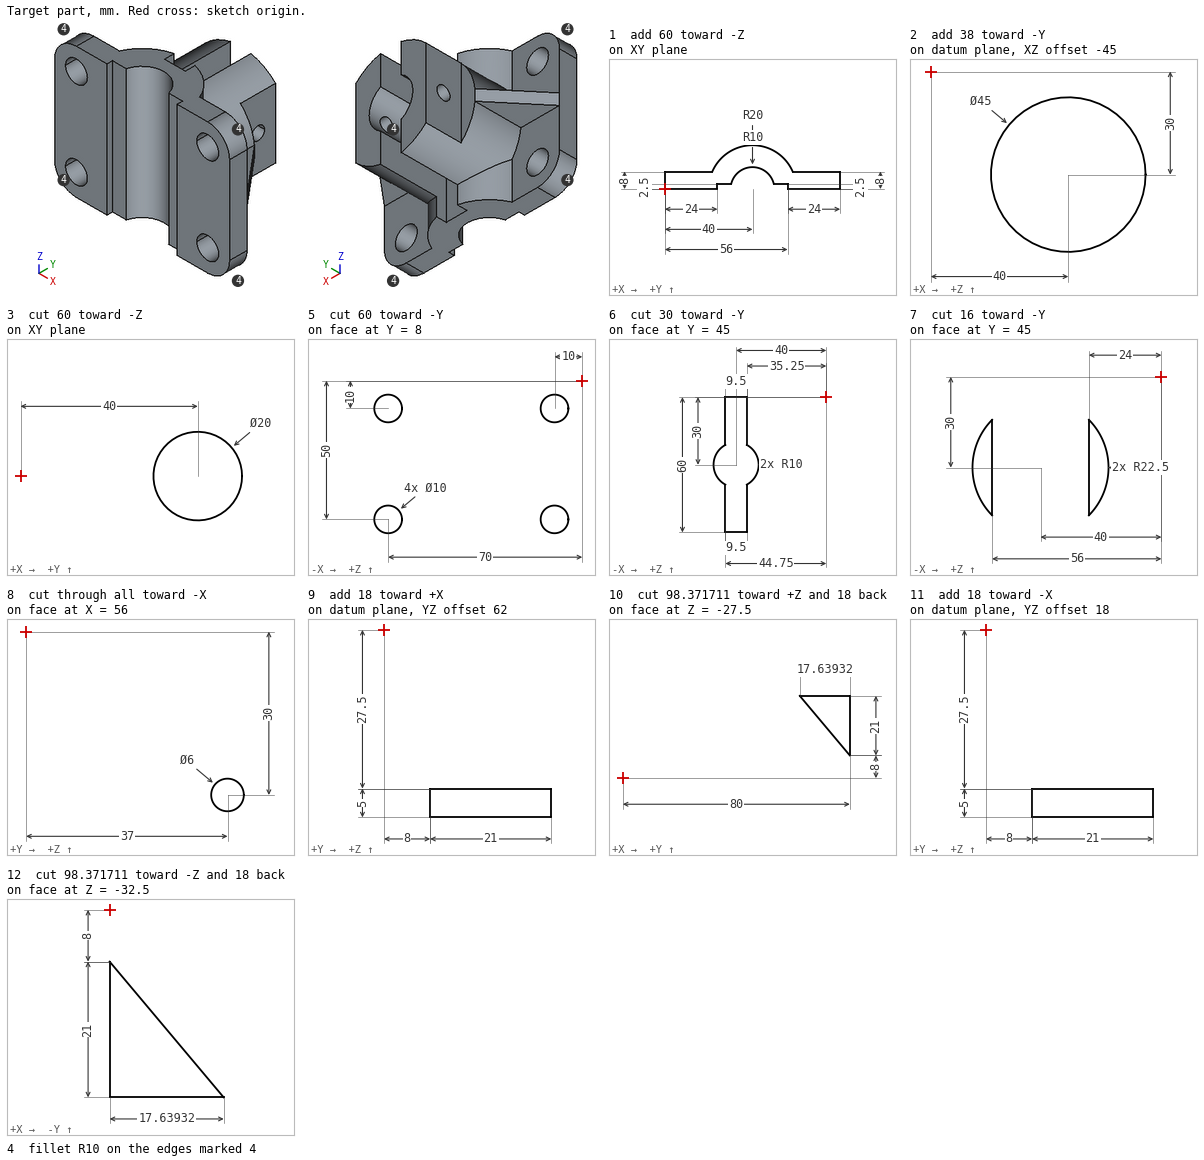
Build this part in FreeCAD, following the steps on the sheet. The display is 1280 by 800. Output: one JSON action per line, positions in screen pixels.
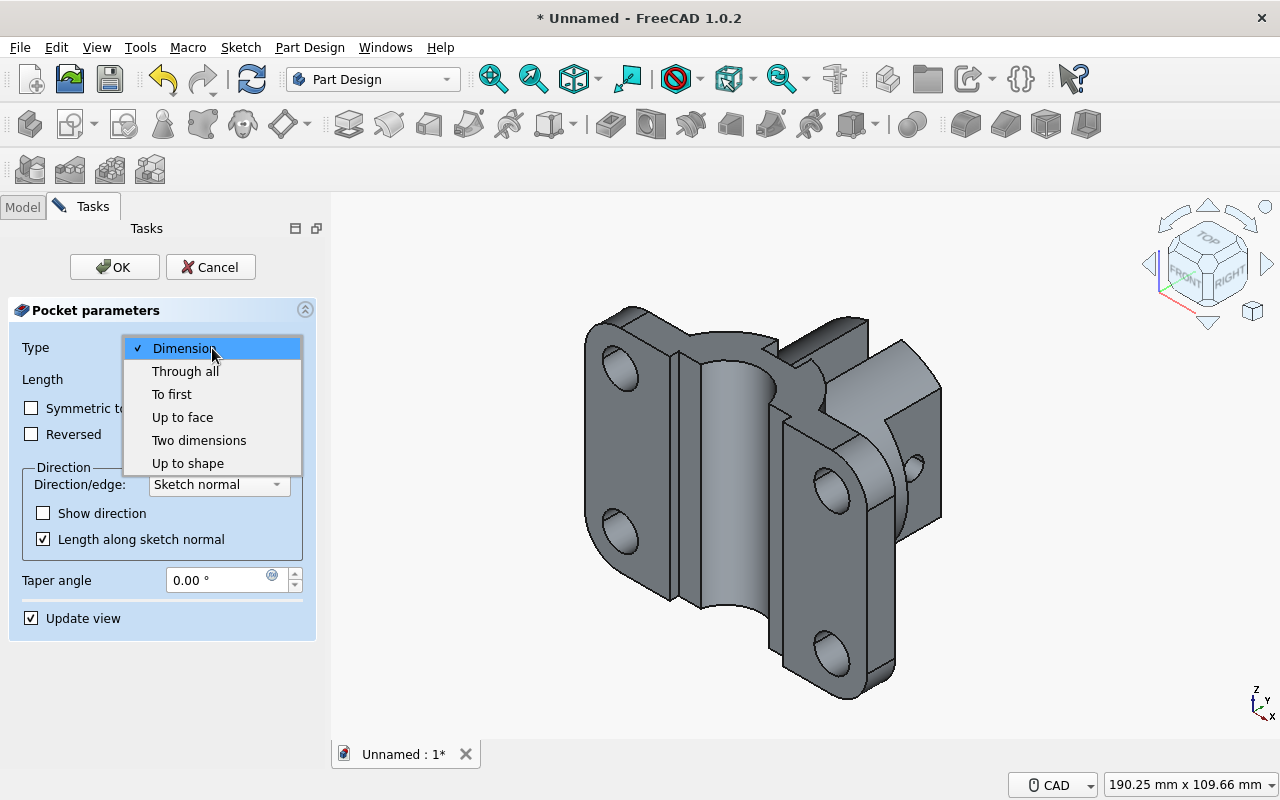
{"action": "left_click", "coordinate": [212, 372]}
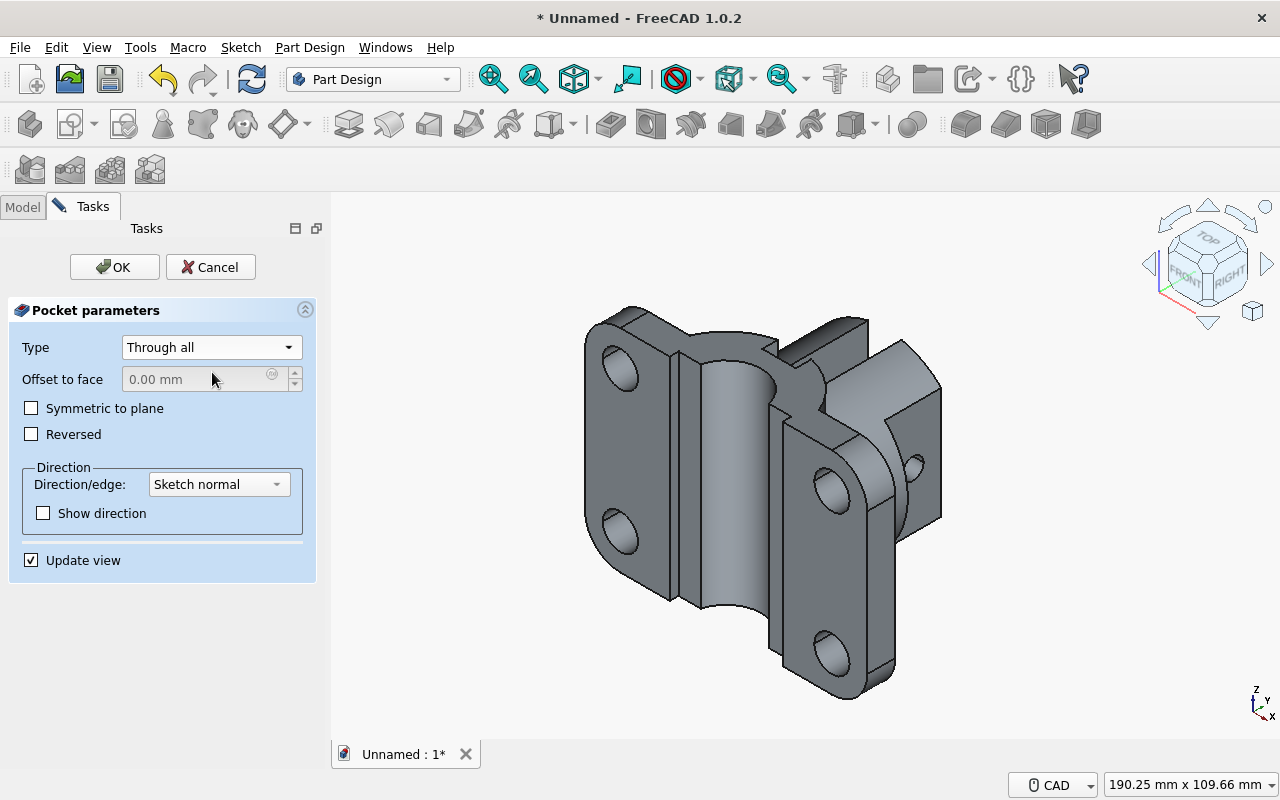
{"action": "left_click", "coordinate": [115, 267]}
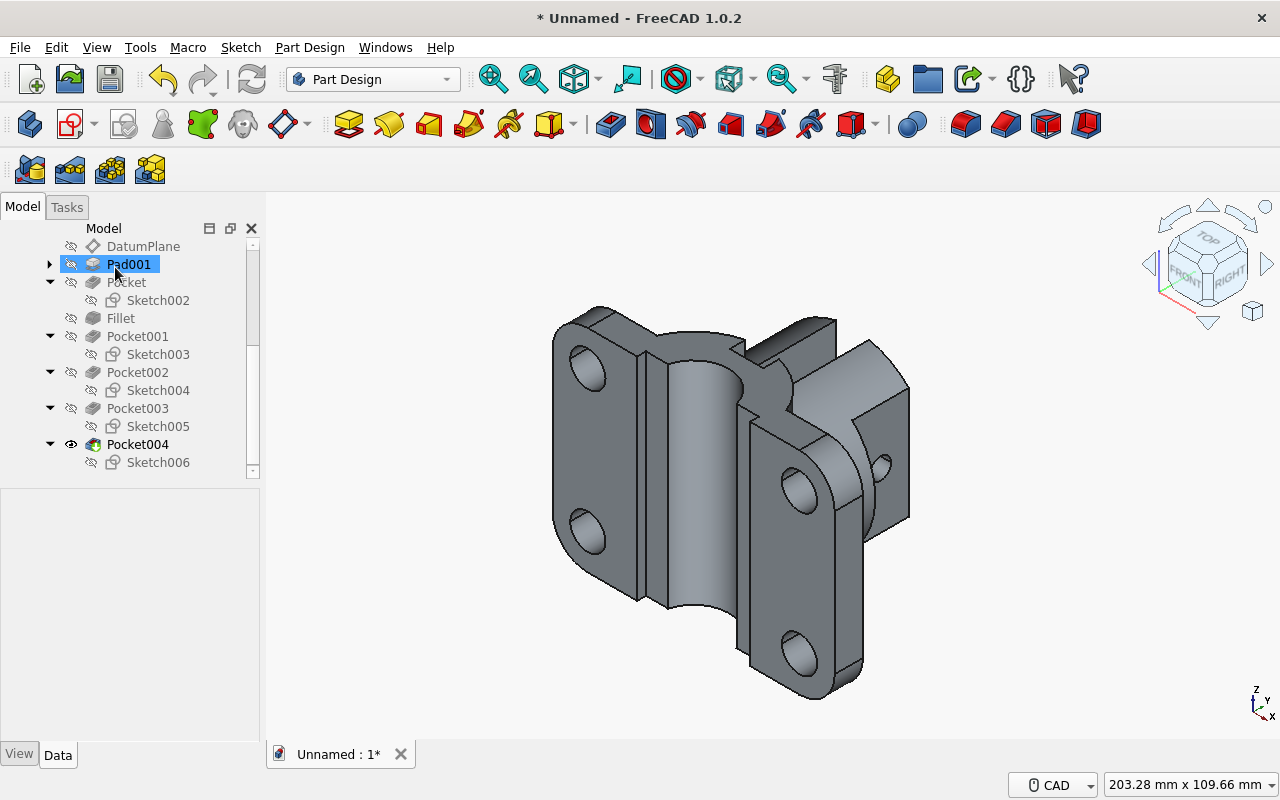
{"action": "scroll", "coordinate": [140, 350], "scroll_direction": "down", "scroll_amount": 3}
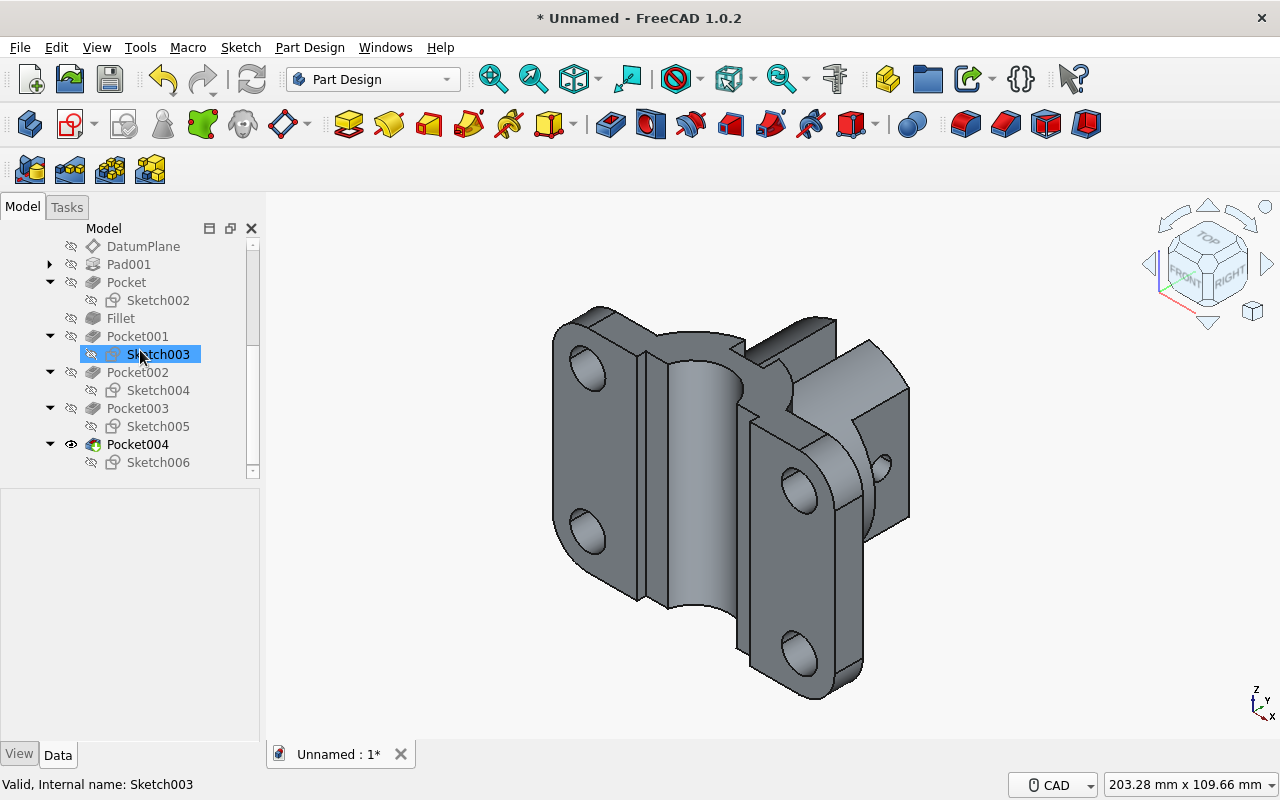
{"action": "scroll", "coordinate": [140, 350], "scroll_direction": "up", "scroll_amount": 15}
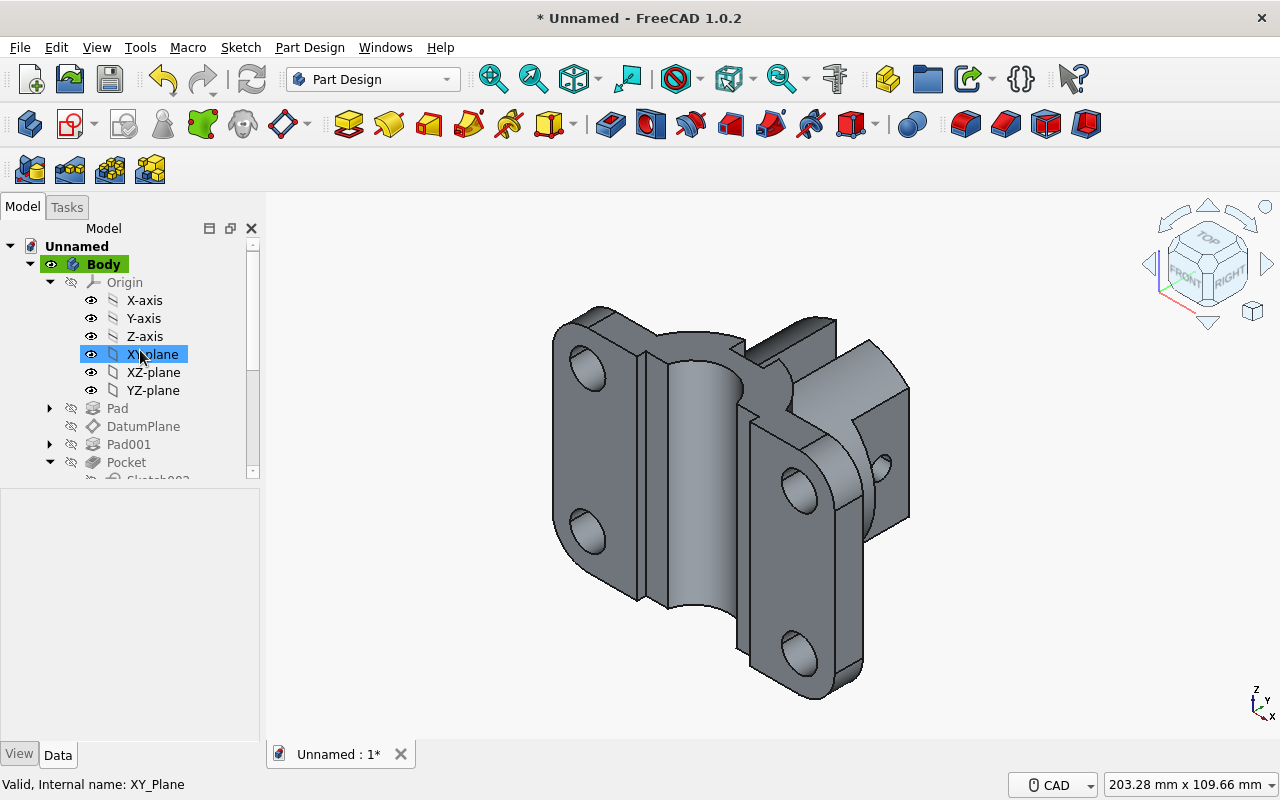
{"action": "left_click", "coordinate": [136, 390]}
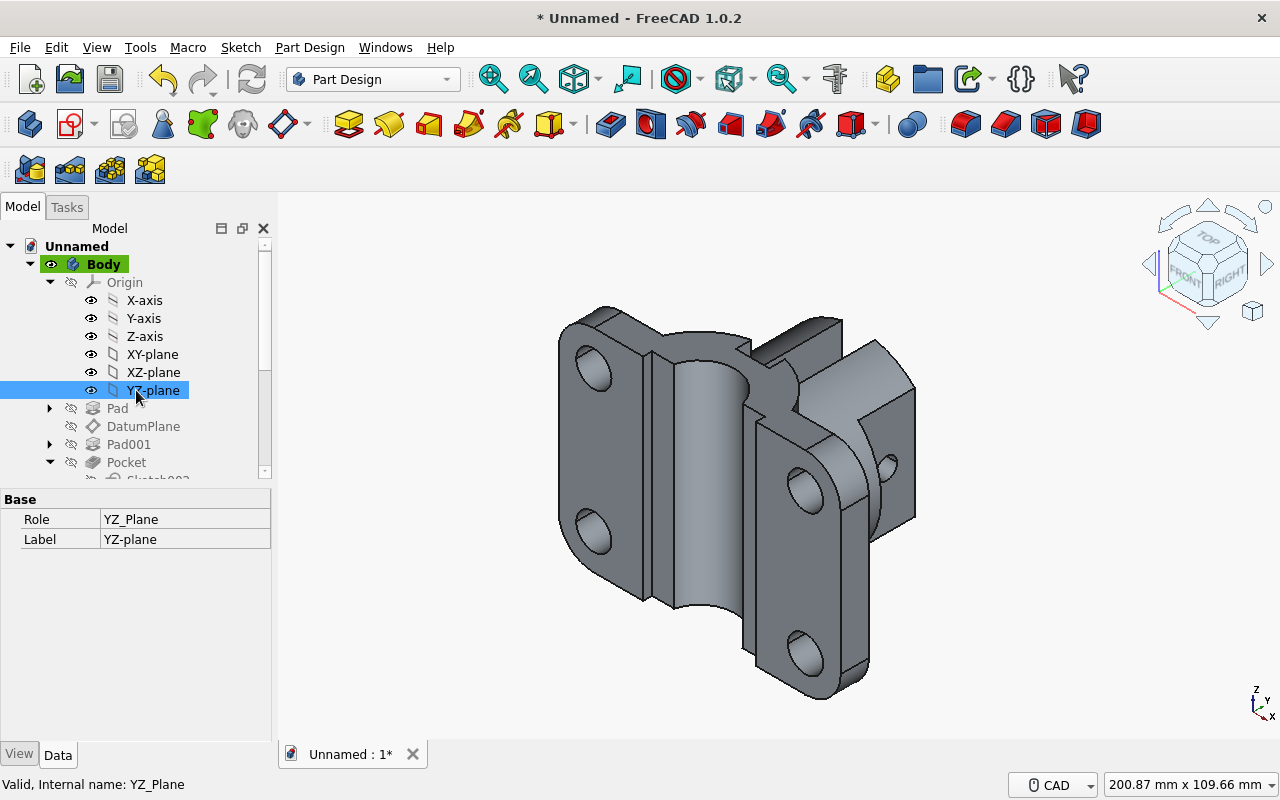
{"action": "left_click", "coordinate": [284, 124]}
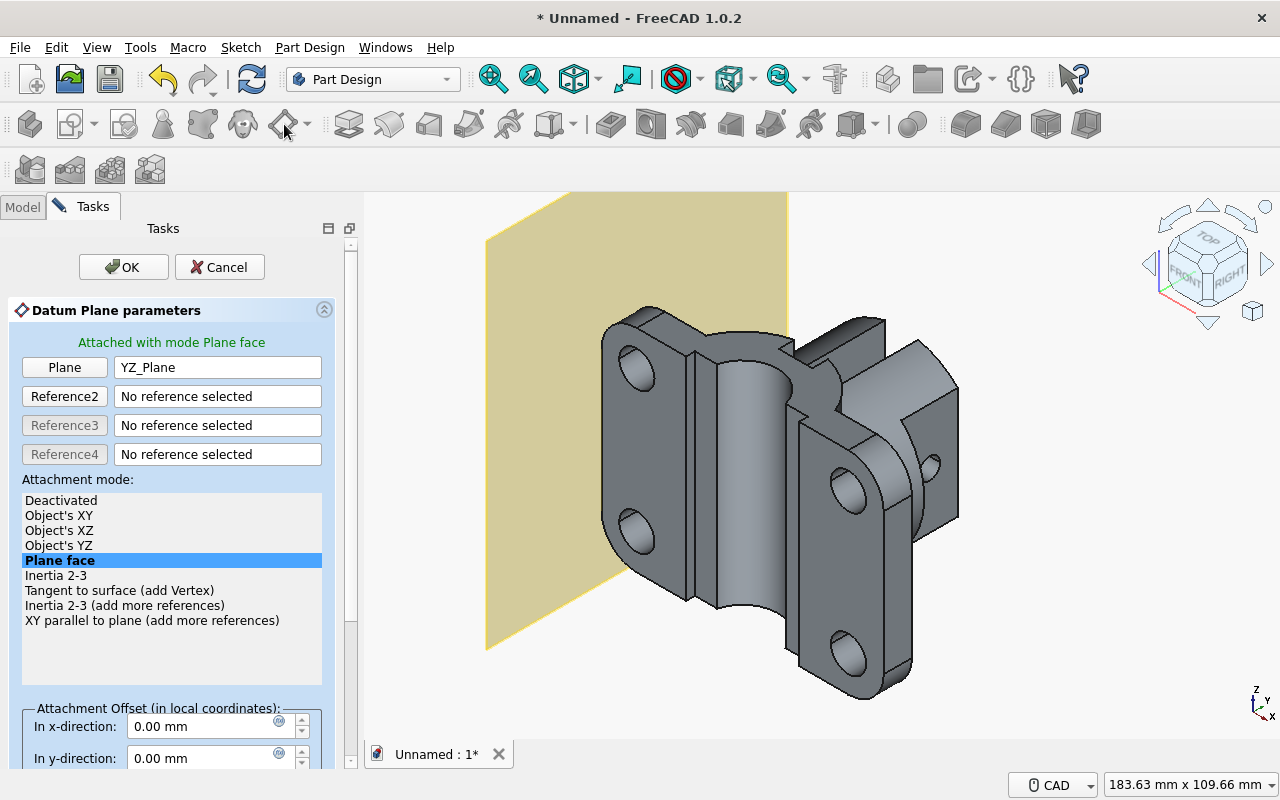
{"action": "scroll", "coordinate": [351, 503], "scroll_direction": "down", "scroll_amount": 2}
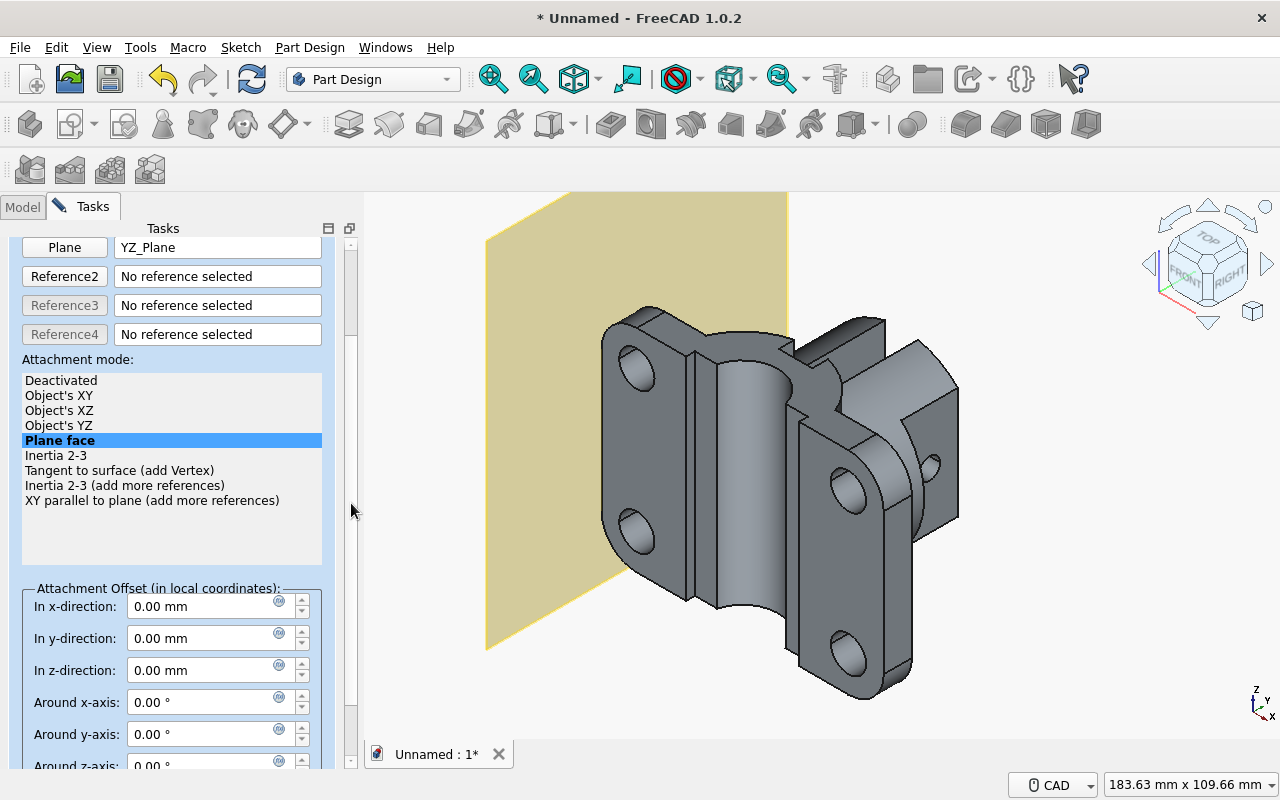
{"action": "triple_click", "coordinate": [210, 670]}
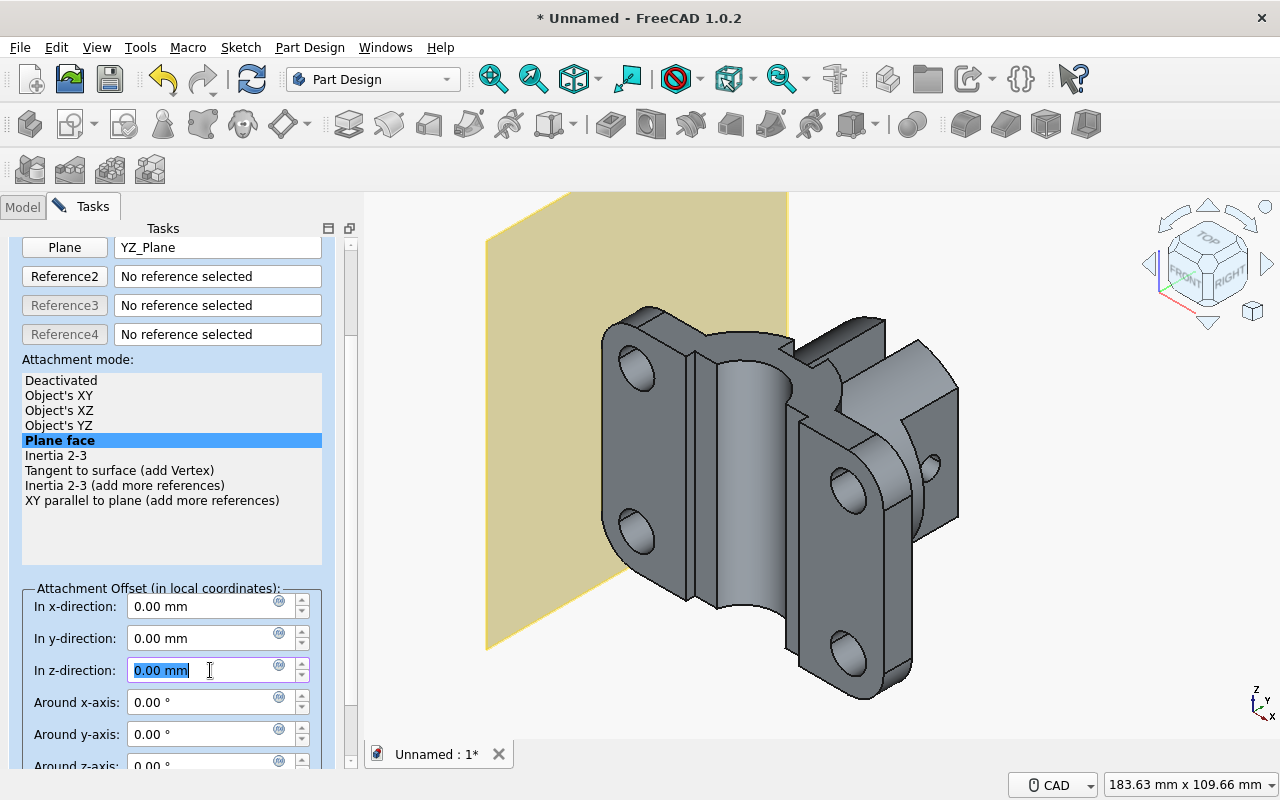
{"action": "type", "text": "62"}
{"action": "key", "text": "Tab"}